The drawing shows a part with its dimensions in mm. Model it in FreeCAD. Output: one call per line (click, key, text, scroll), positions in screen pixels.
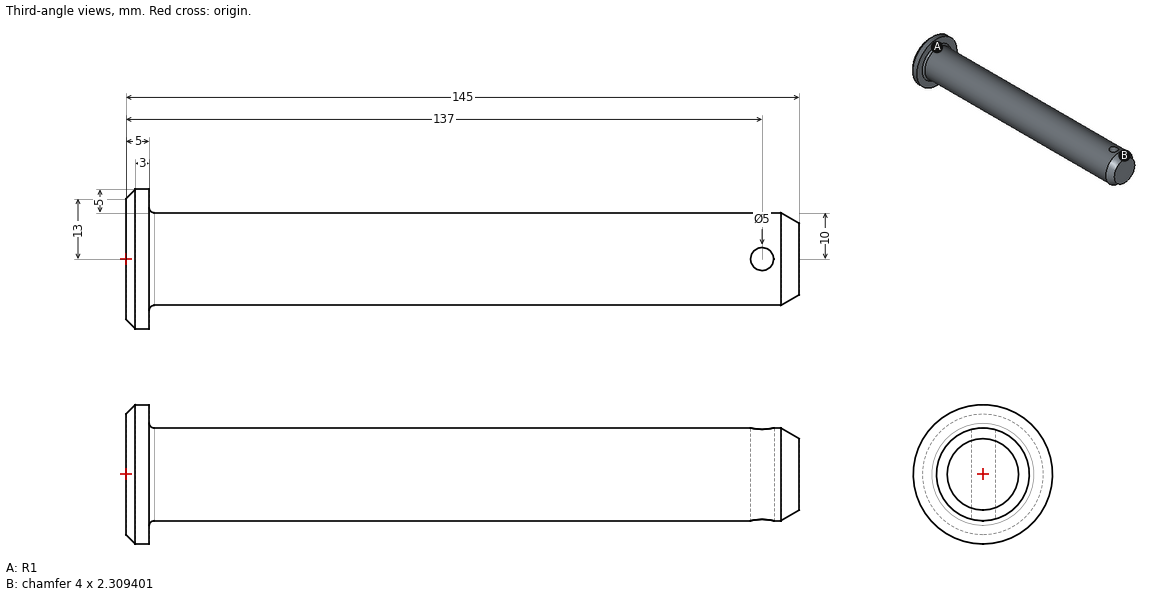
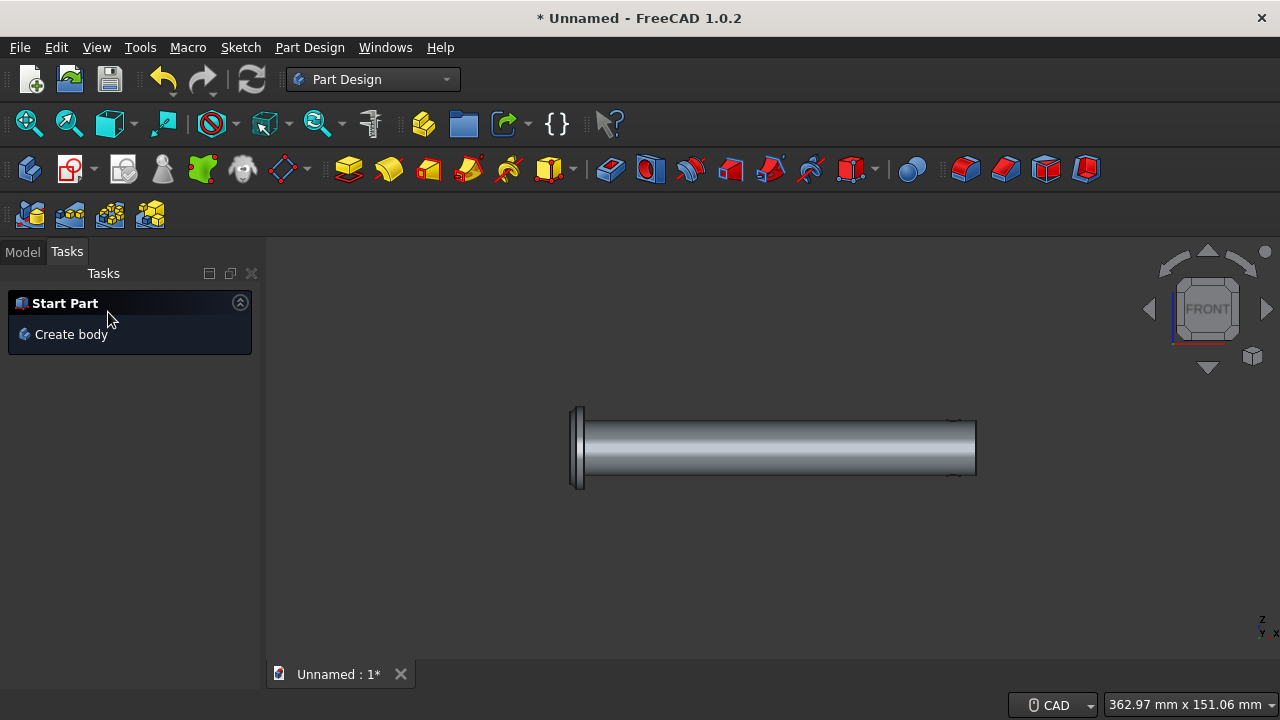
key(v)
key(f)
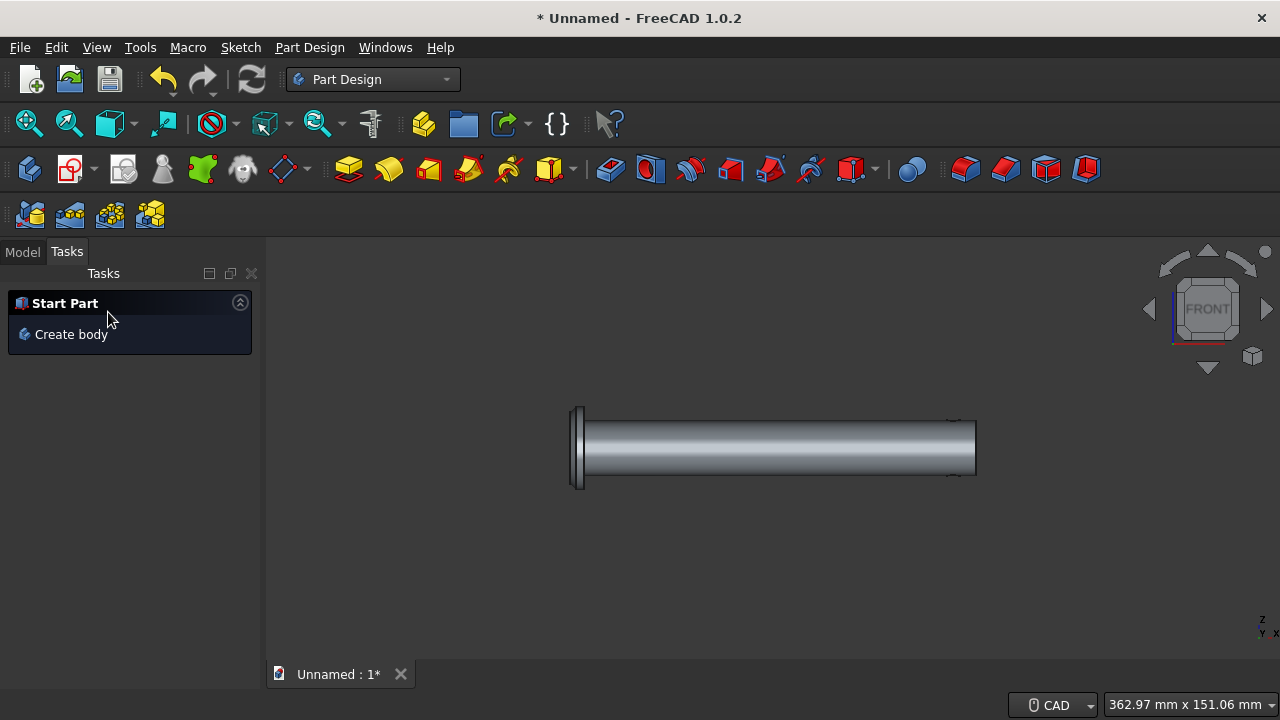
key(3)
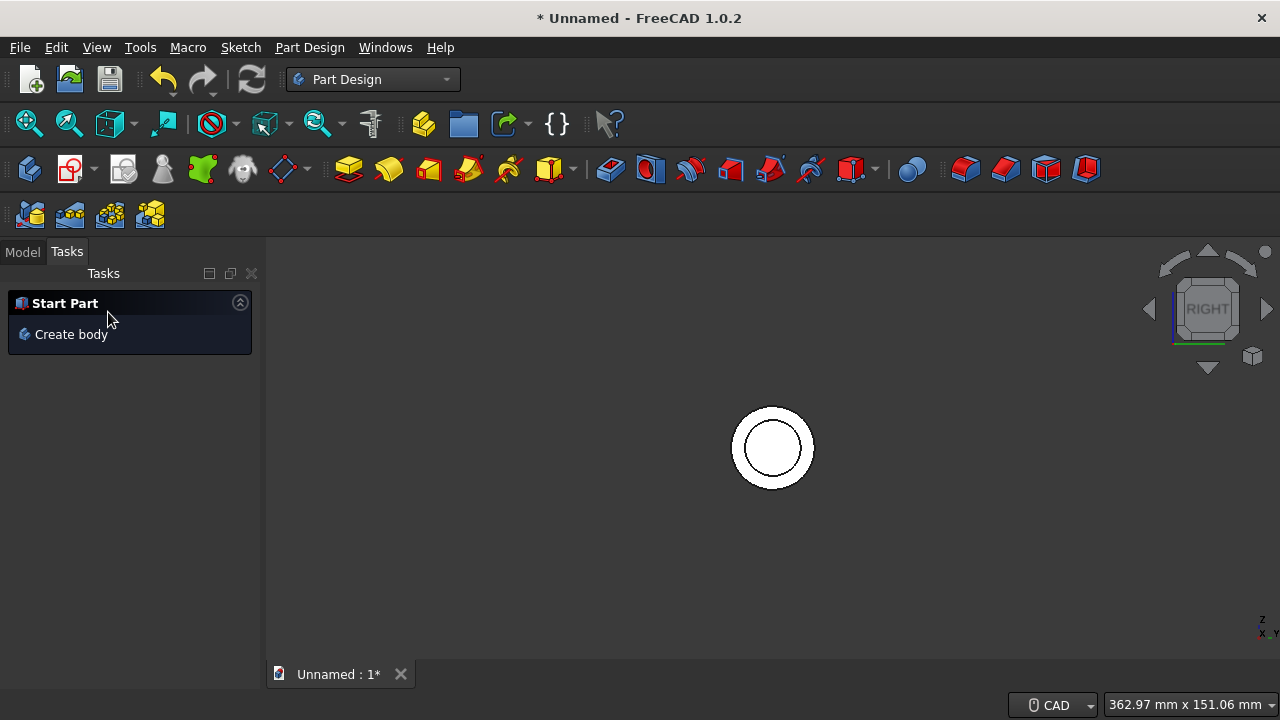
click(30, 124)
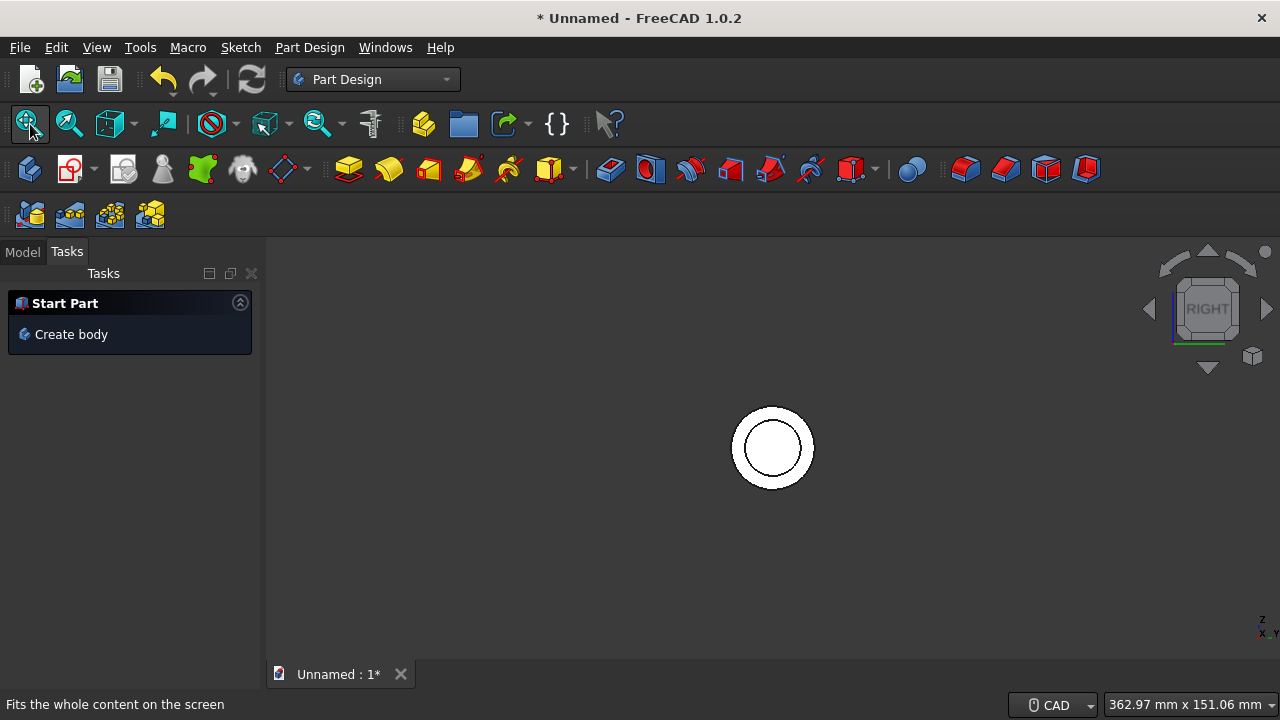
key(5)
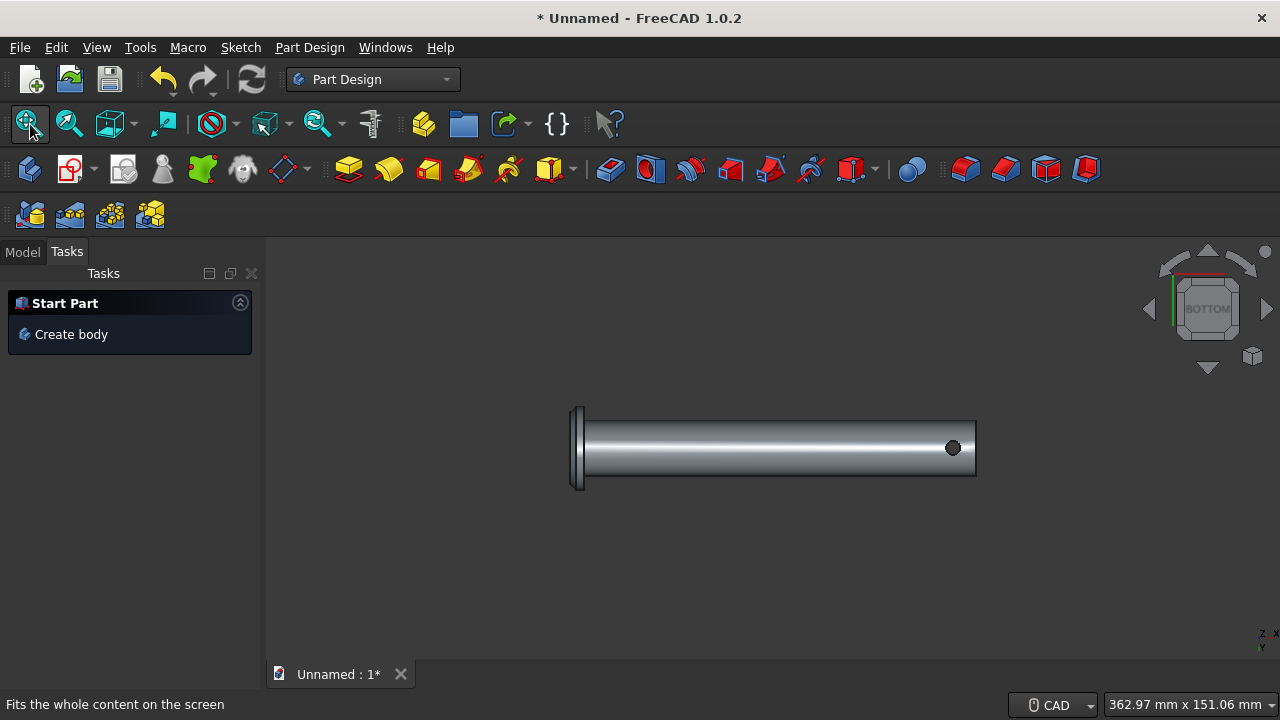
key(v)
key(f)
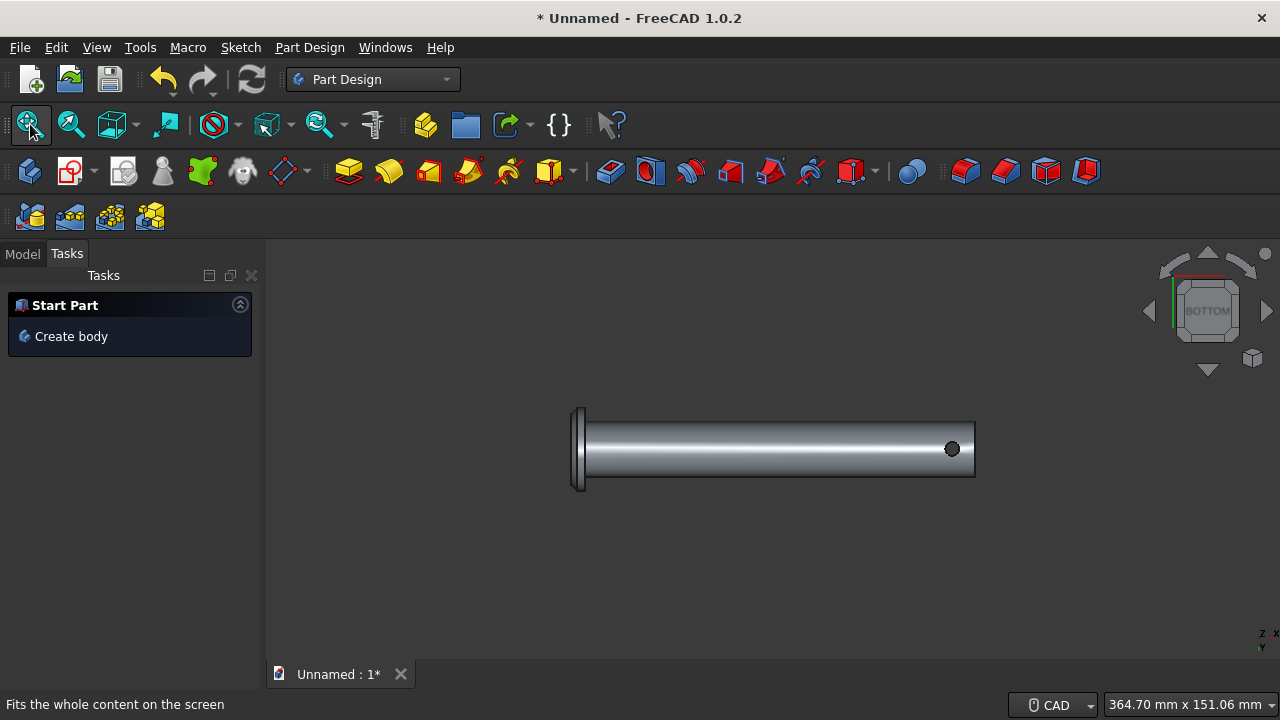
key(4)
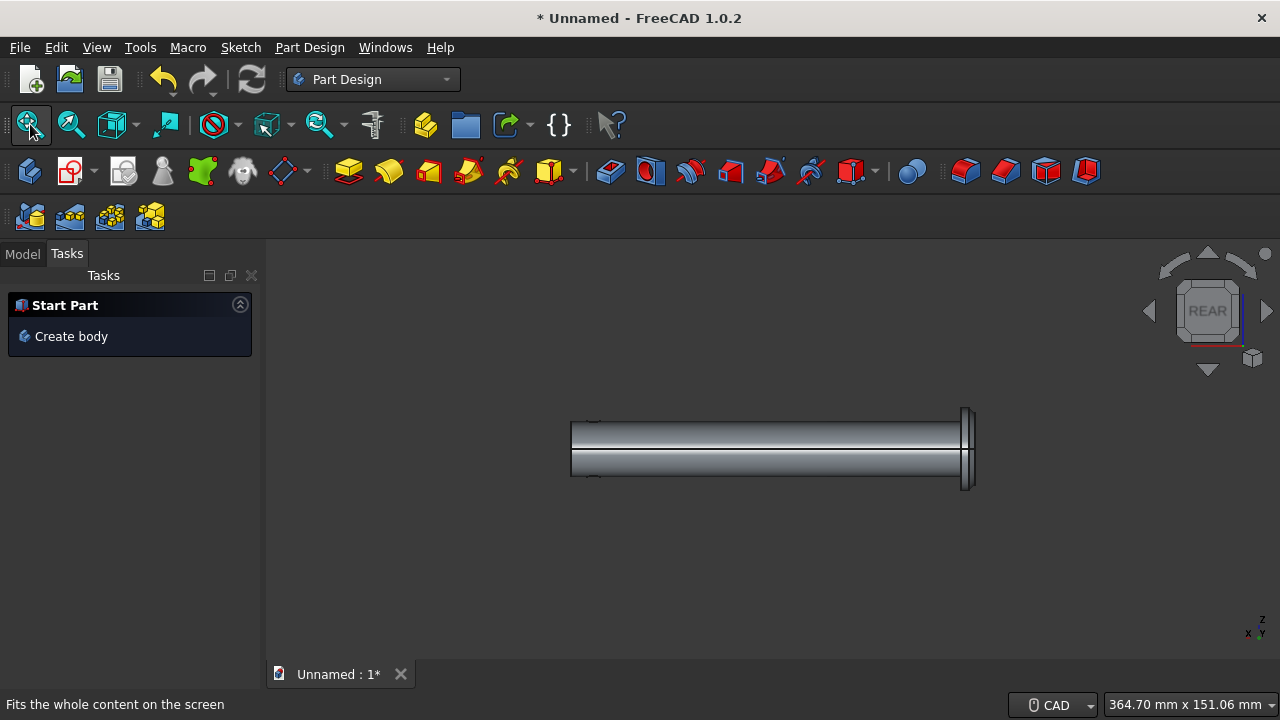
click(32, 126)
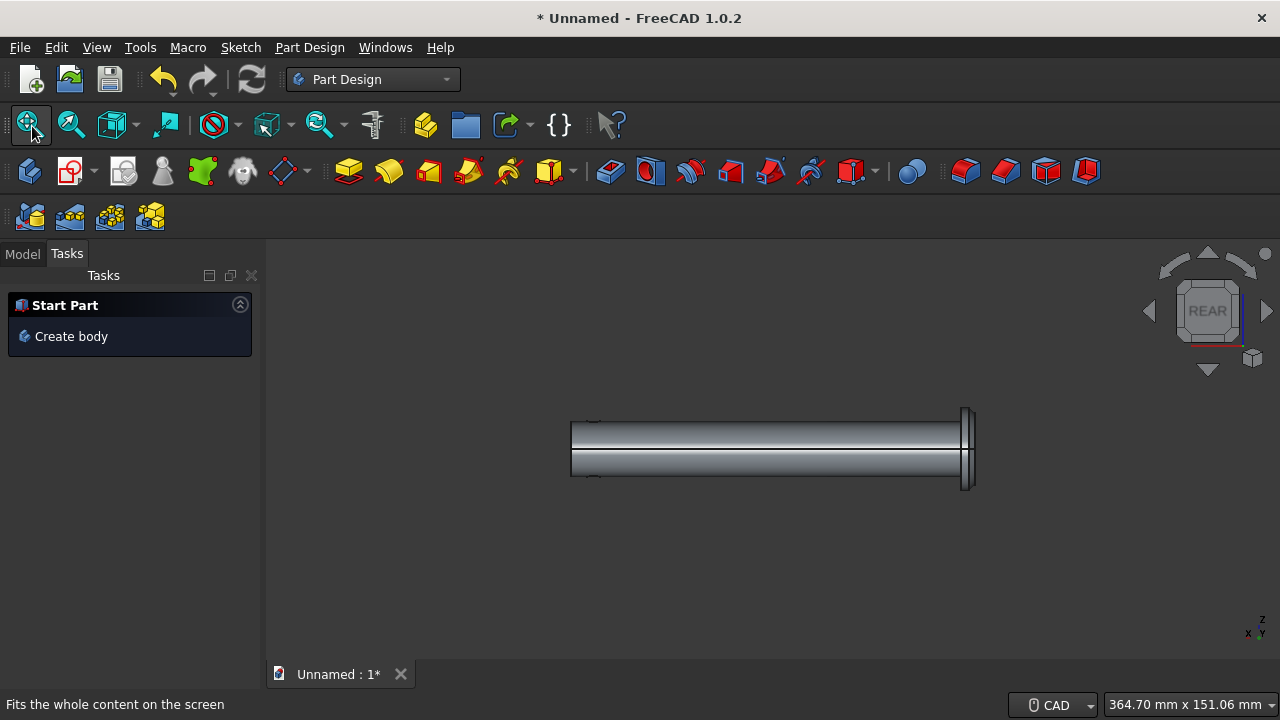
key(6)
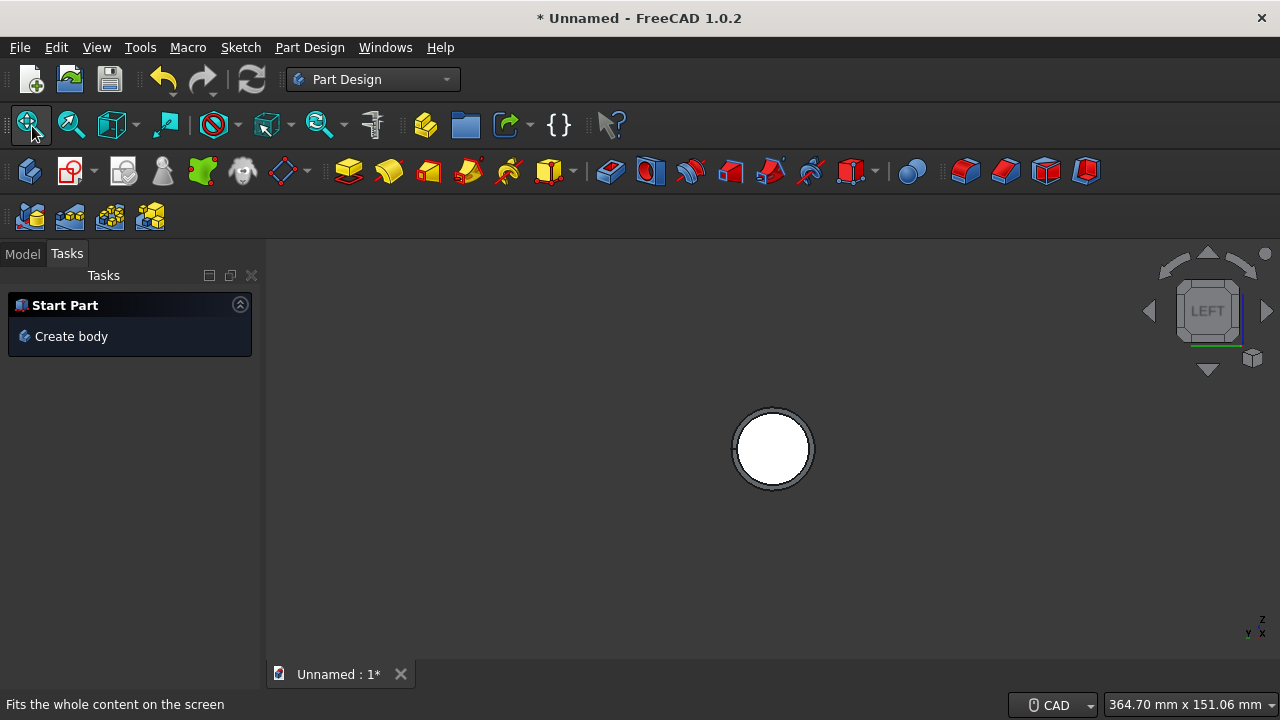
key(v)
key(f)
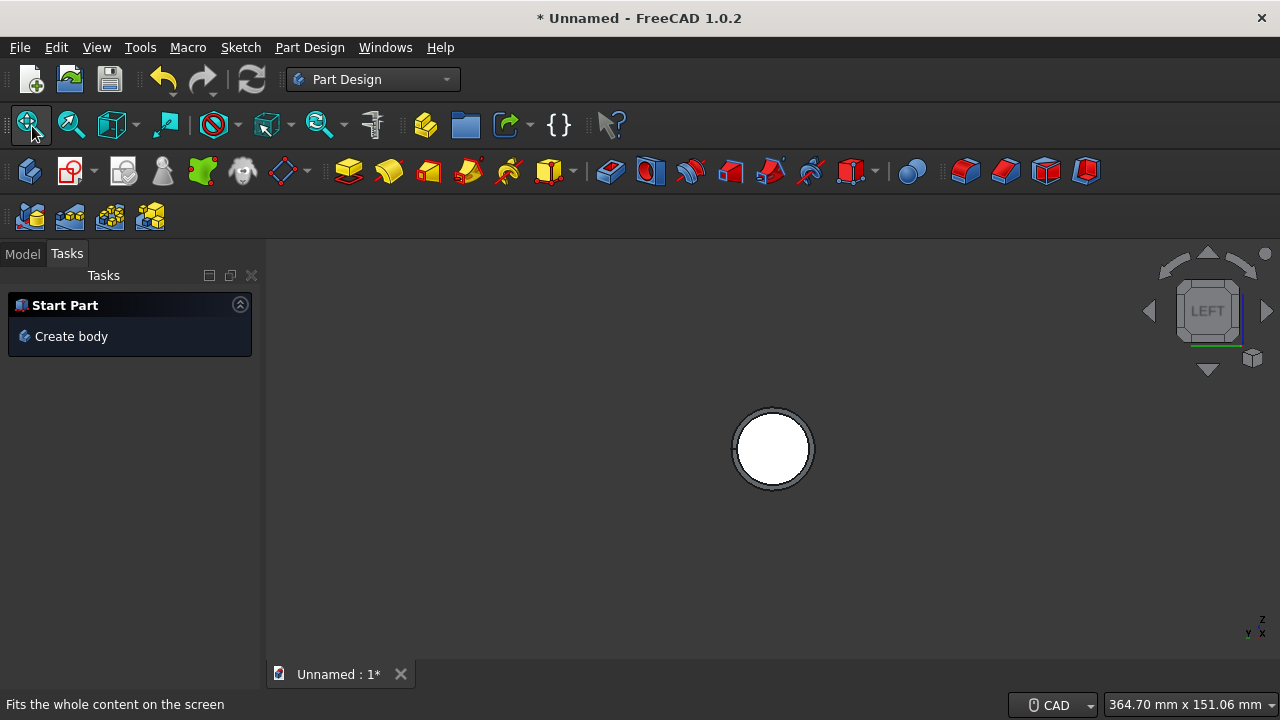
key(v)
key(3)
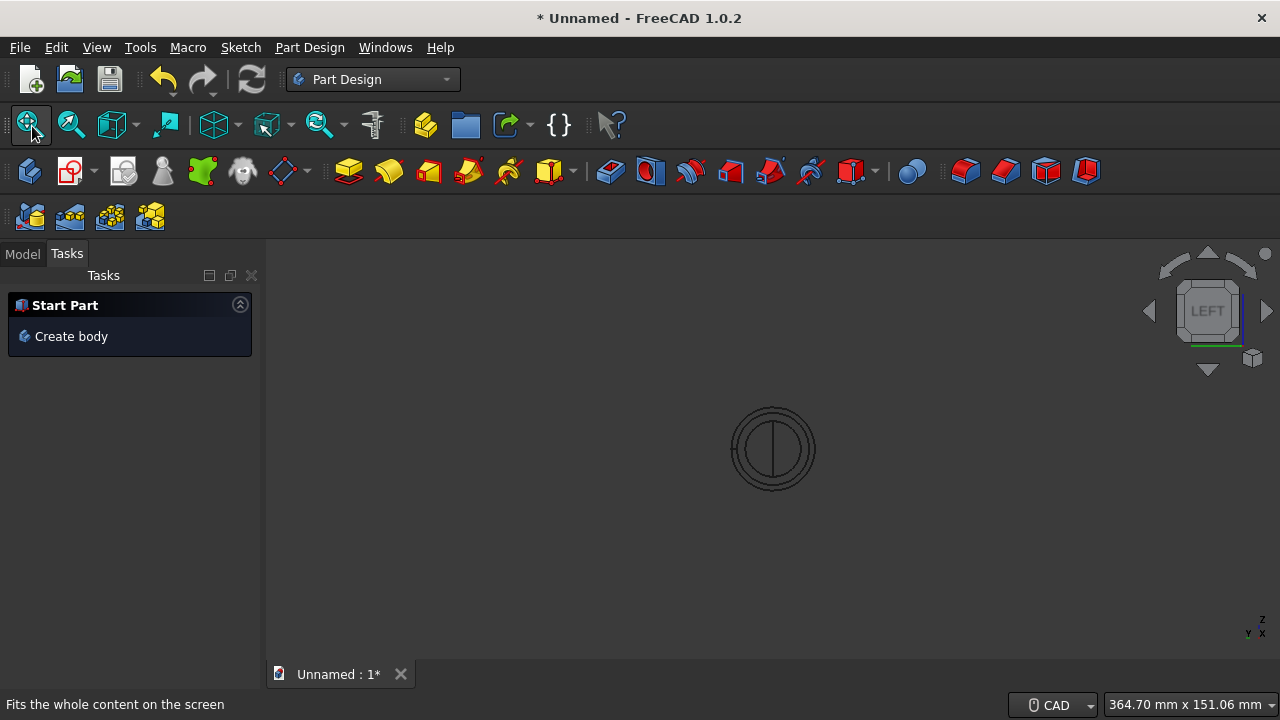
key(0)